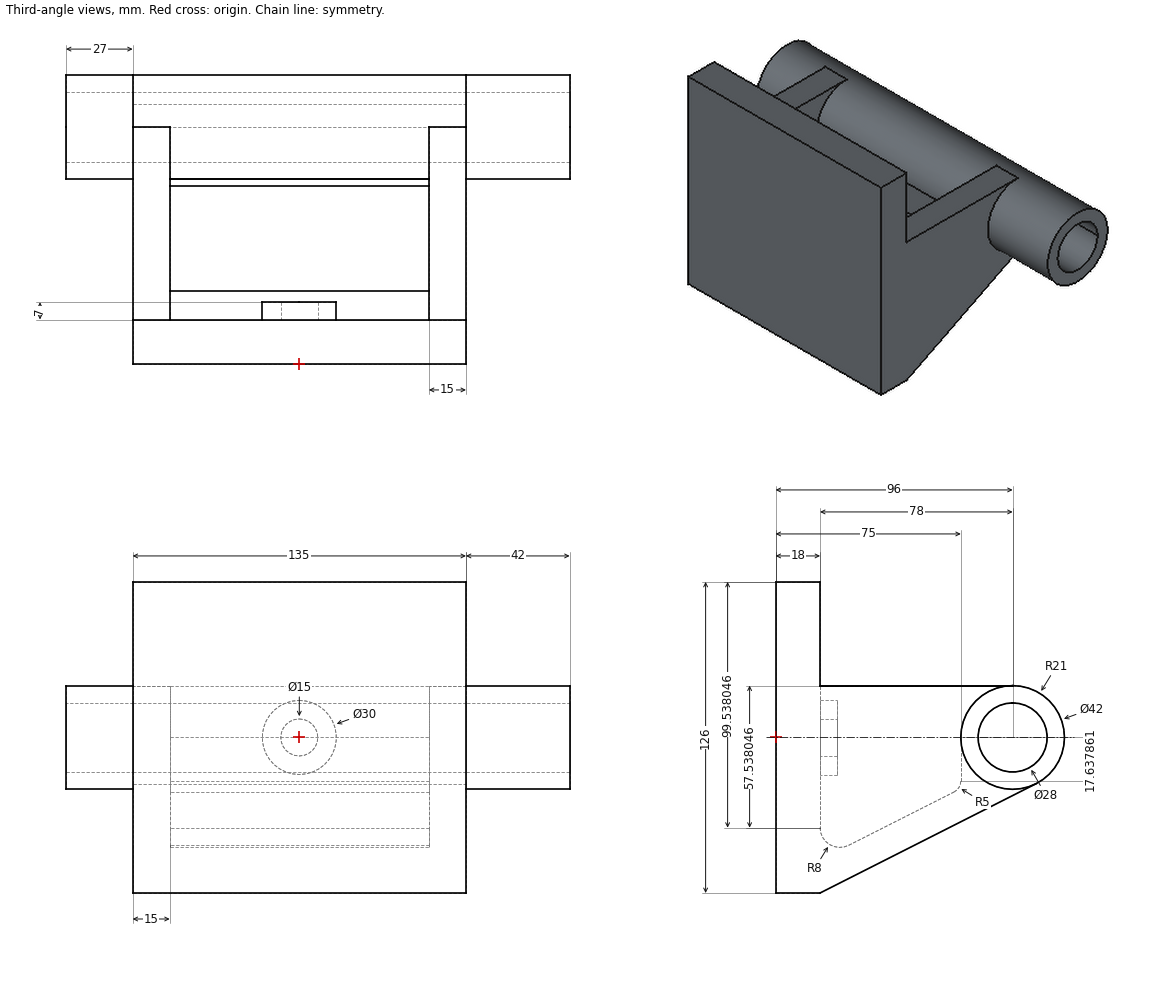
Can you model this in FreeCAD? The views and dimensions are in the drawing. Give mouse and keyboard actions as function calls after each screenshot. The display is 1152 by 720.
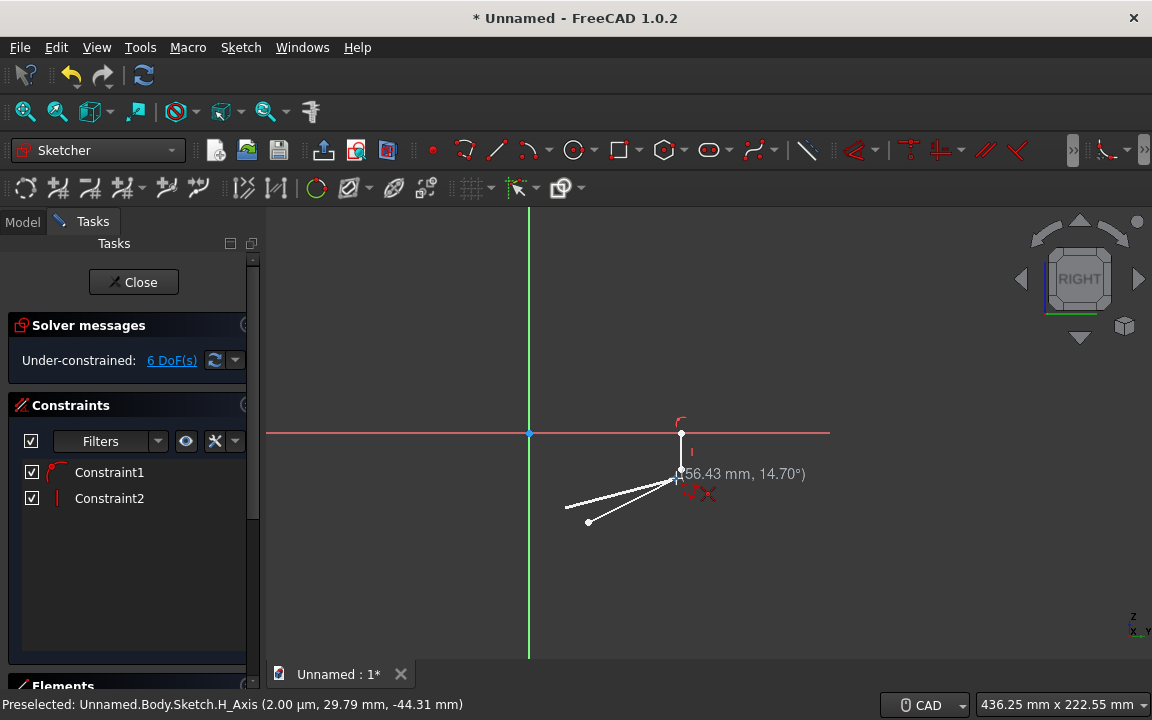
click(565, 305)
click(529, 305)
click(538, 561)
click(566, 561)
click(743, 471)
right_click(743, 471)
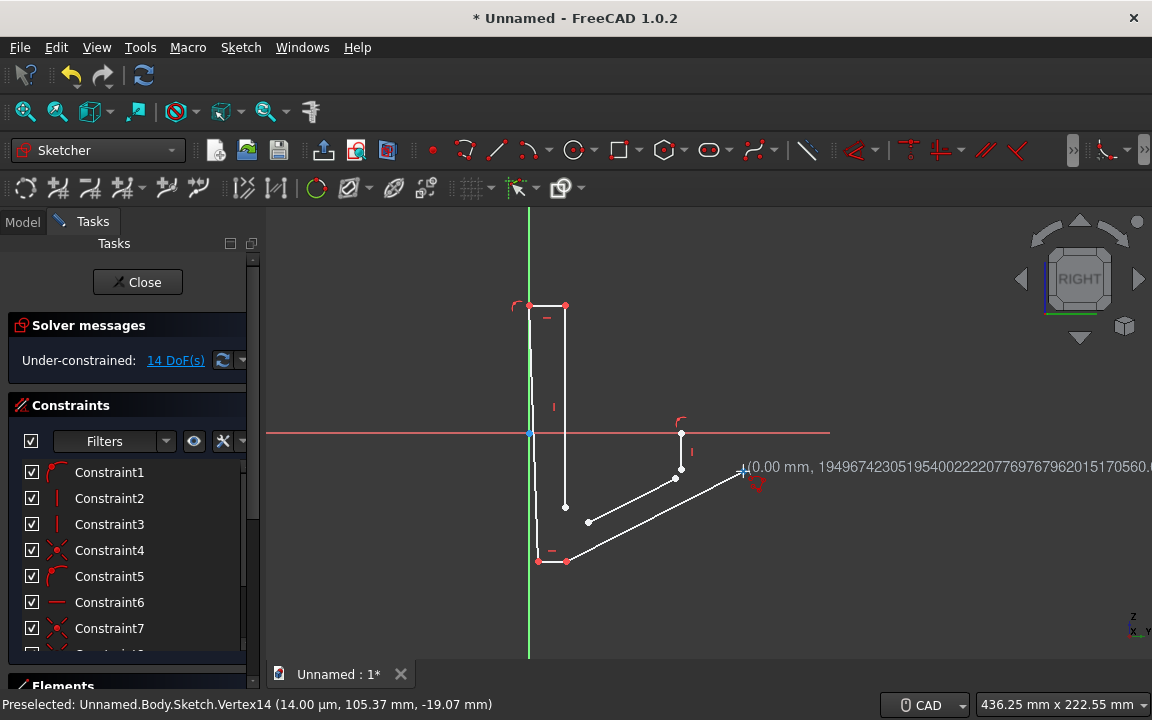
key(g)
key(3)
key(a)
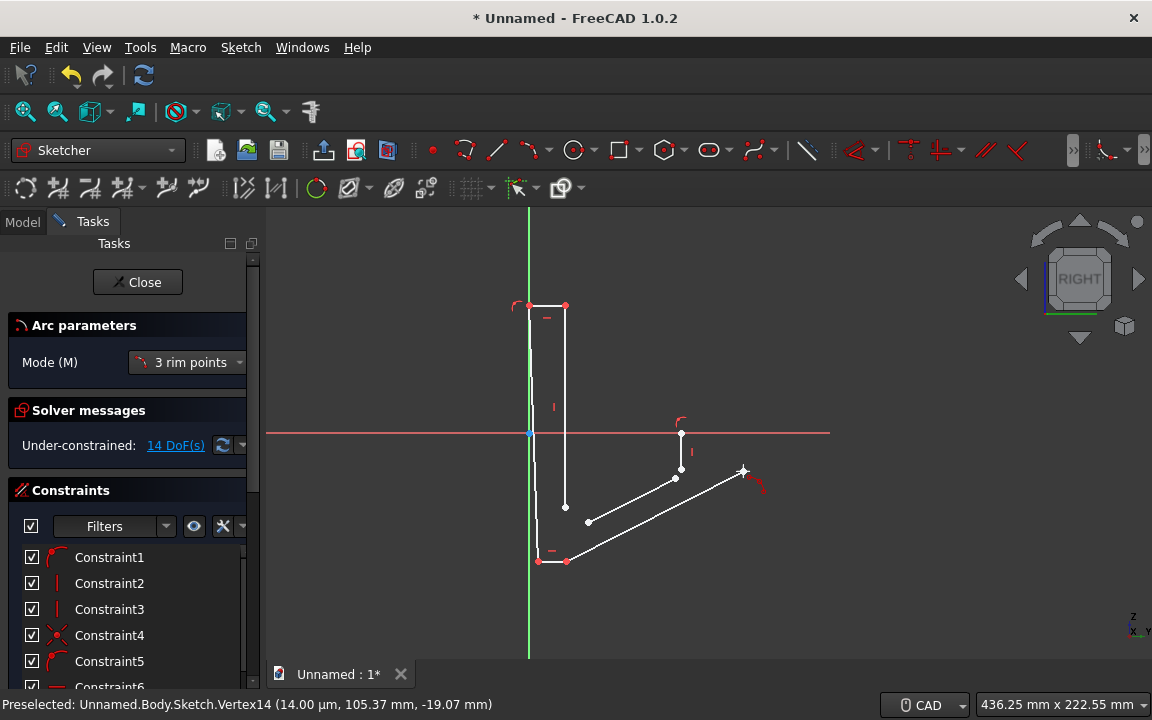
scroll(681, 469, up, 3)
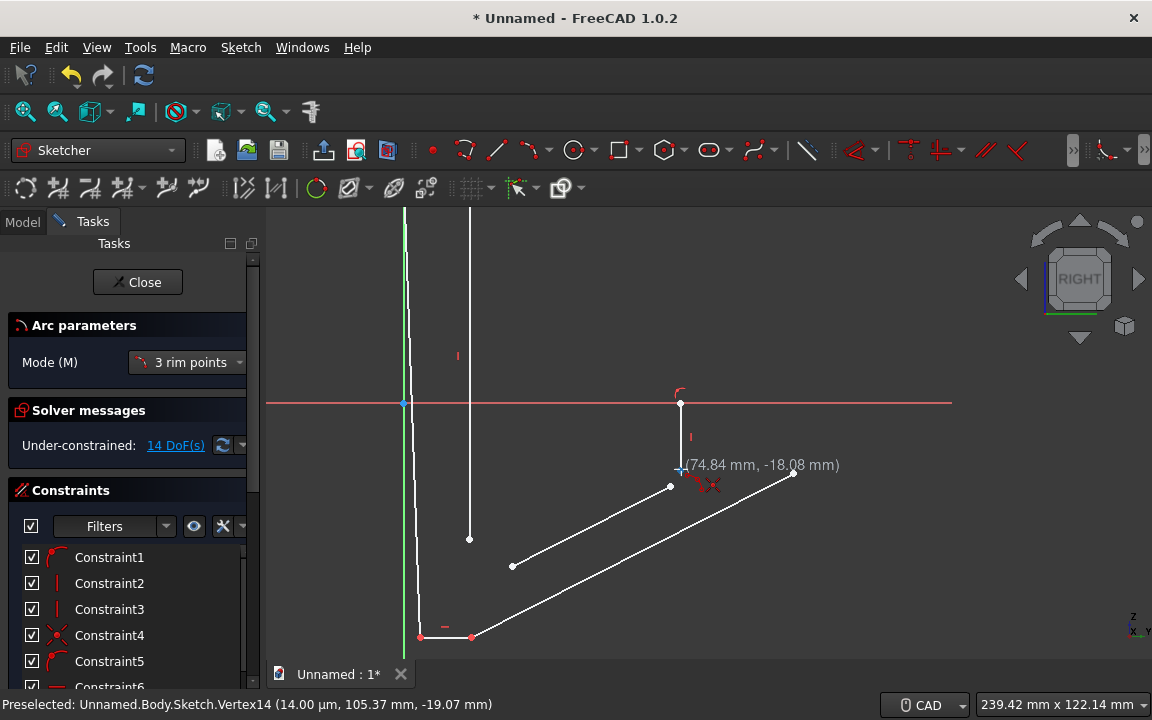
click(681, 470)
click(671, 486)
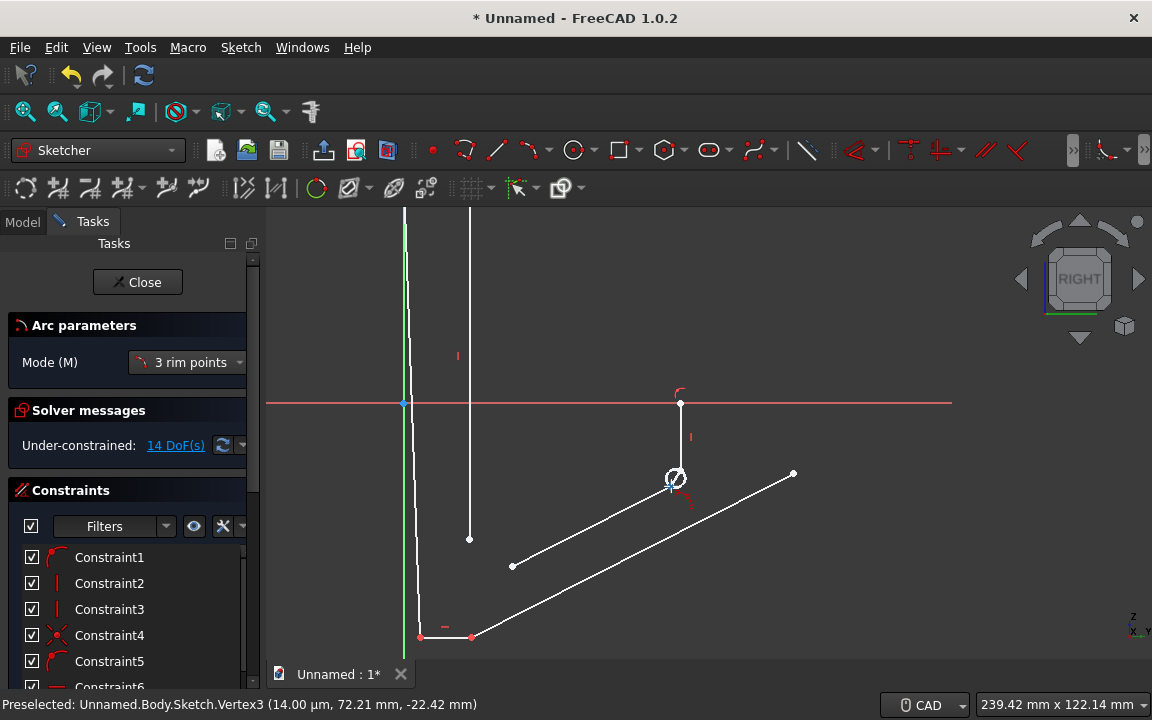
scroll(678, 478, up, 9)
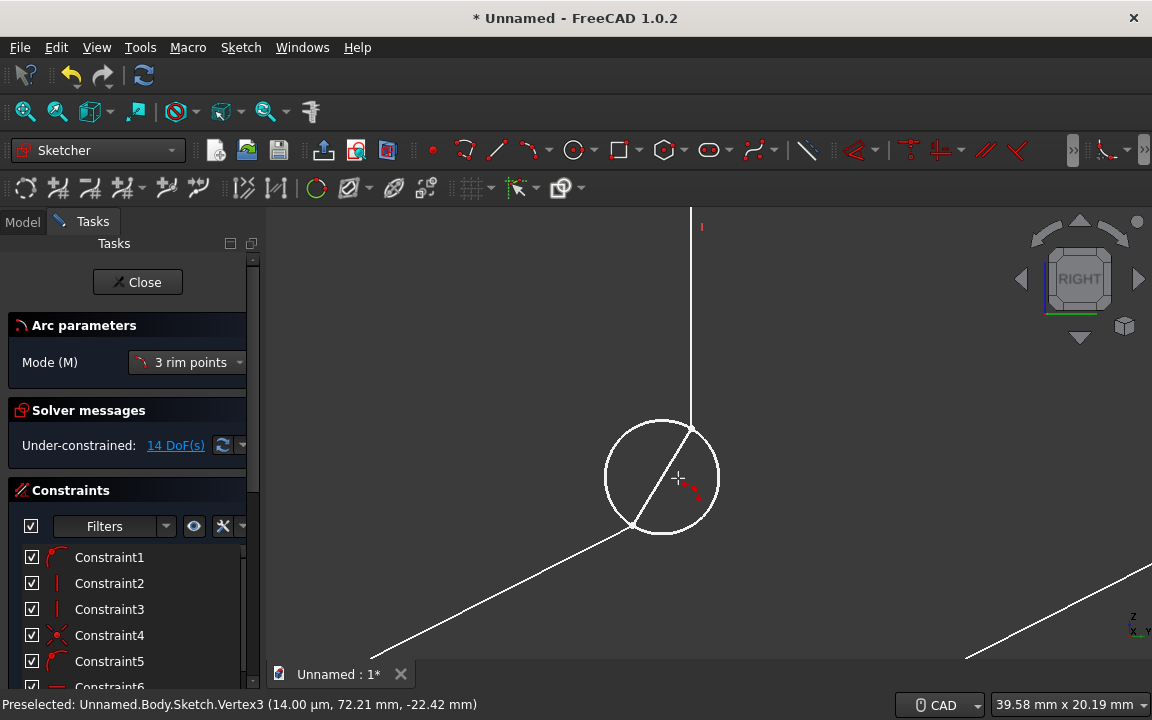
click(678, 477)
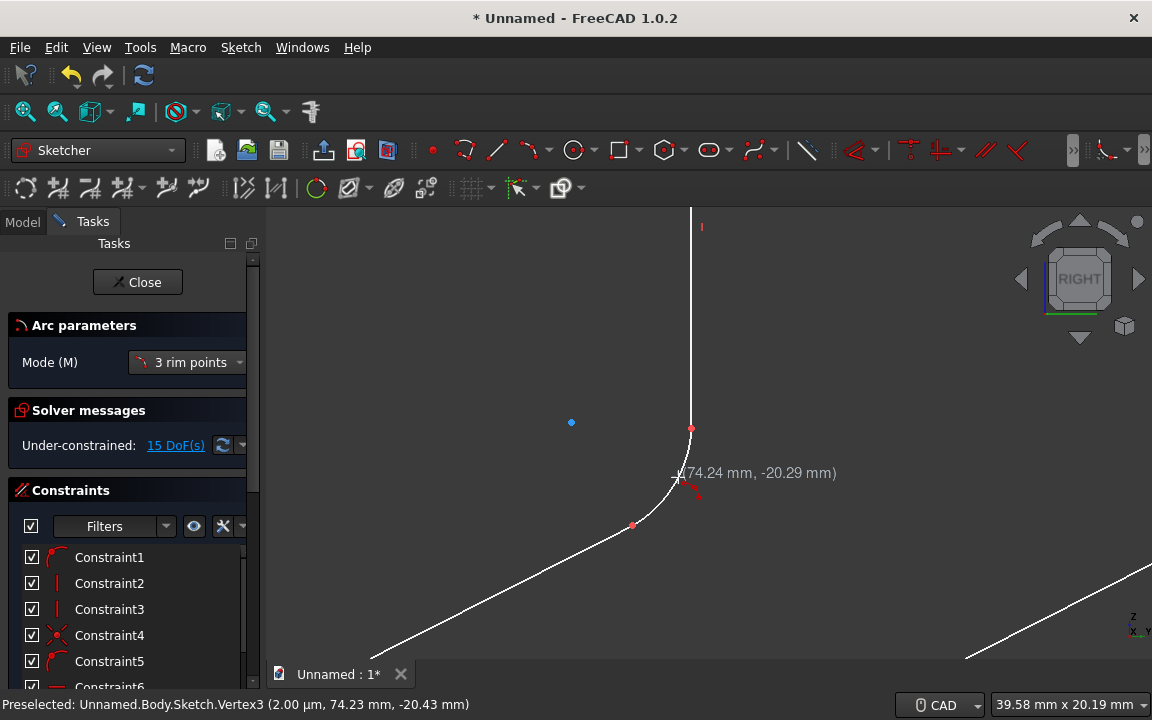
scroll(680, 474, down, 12)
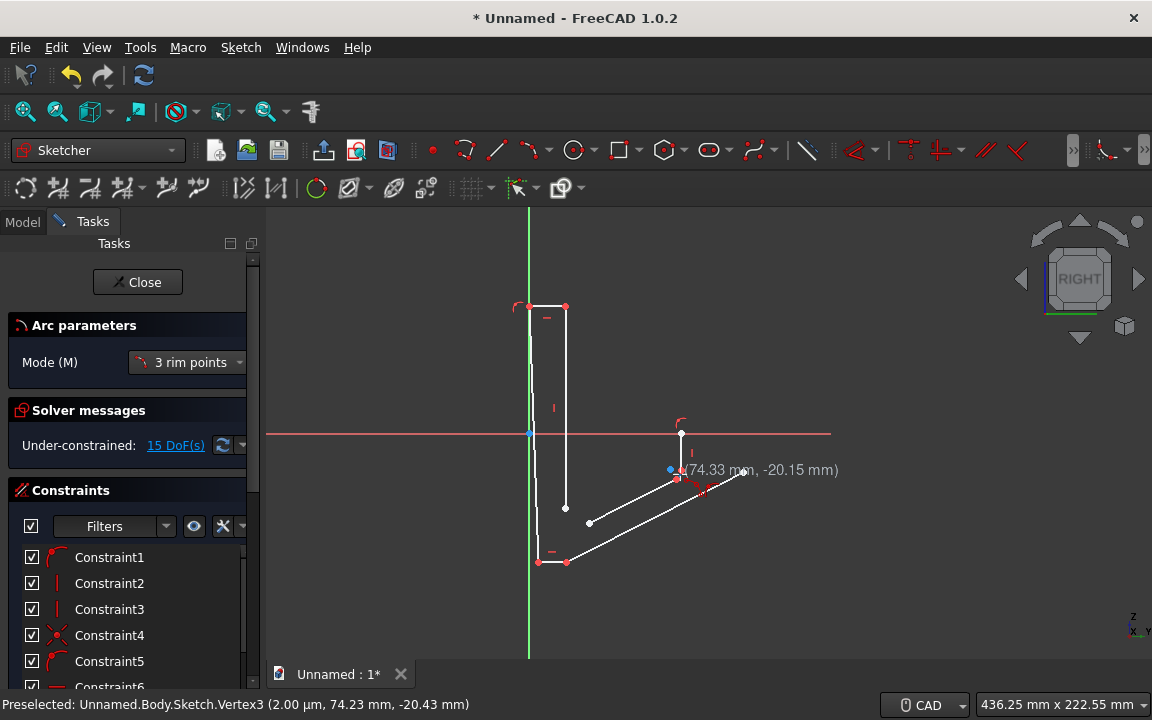
click(589, 523)
click(566, 508)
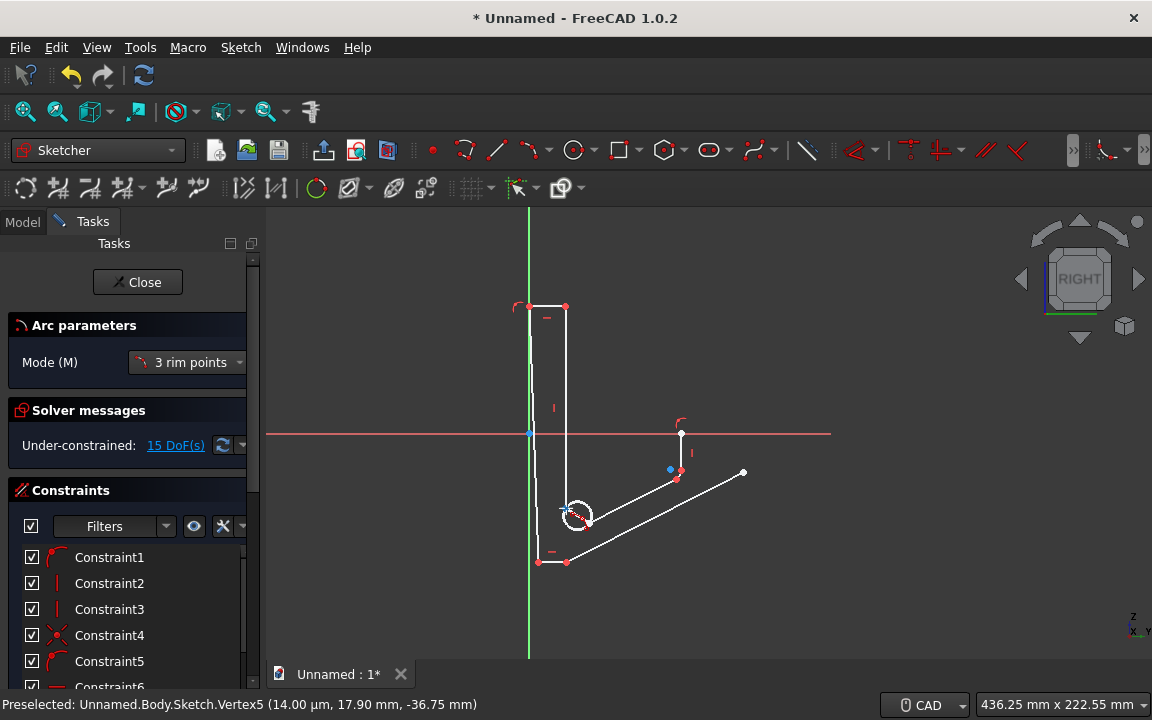
scroll(574, 522, up, 4)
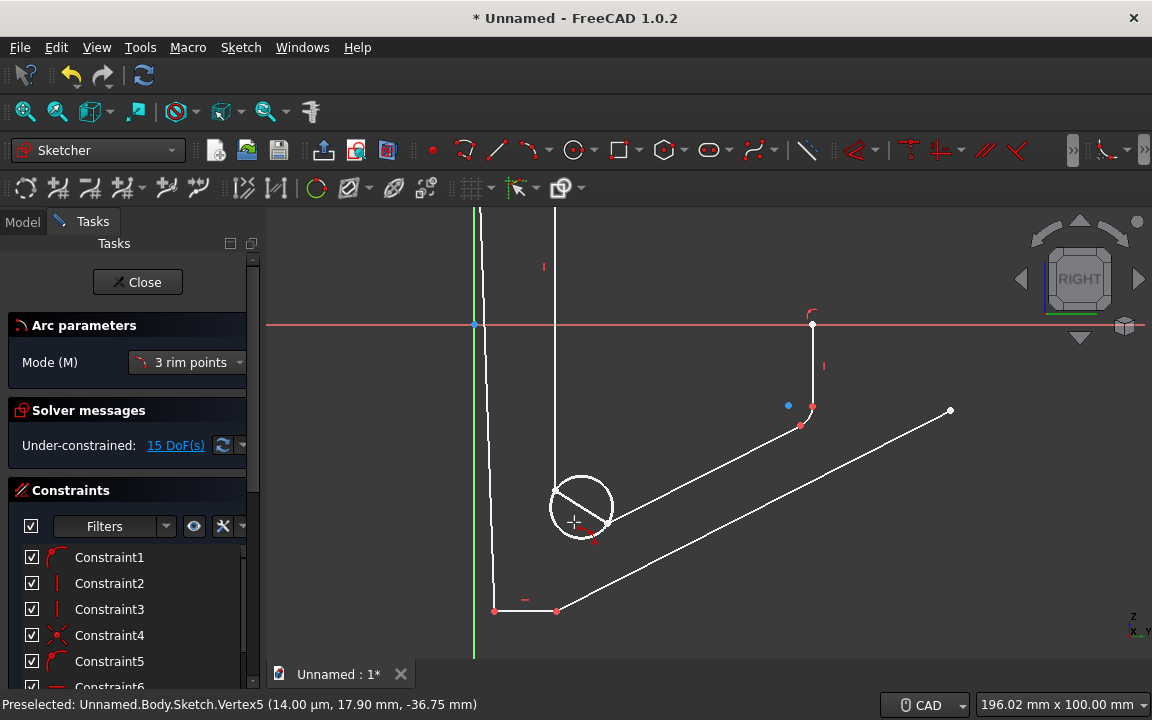
click(573, 521)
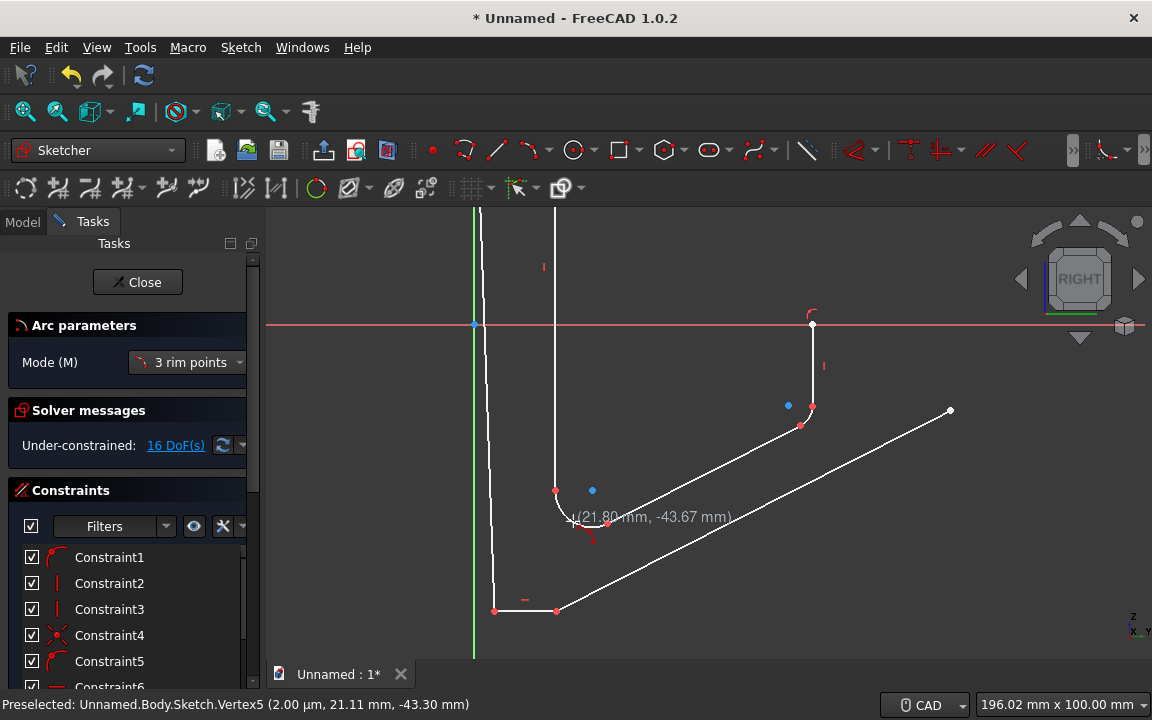
click(951, 411)
click(813, 325)
click(958, 244)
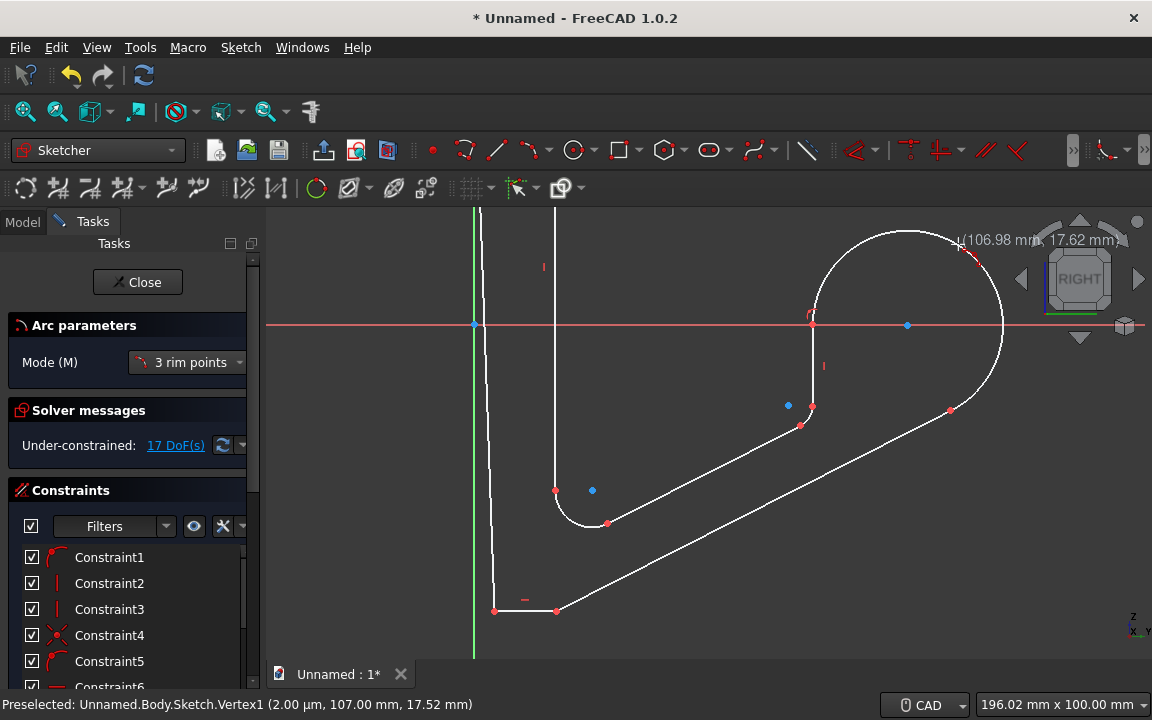
click(574, 150)